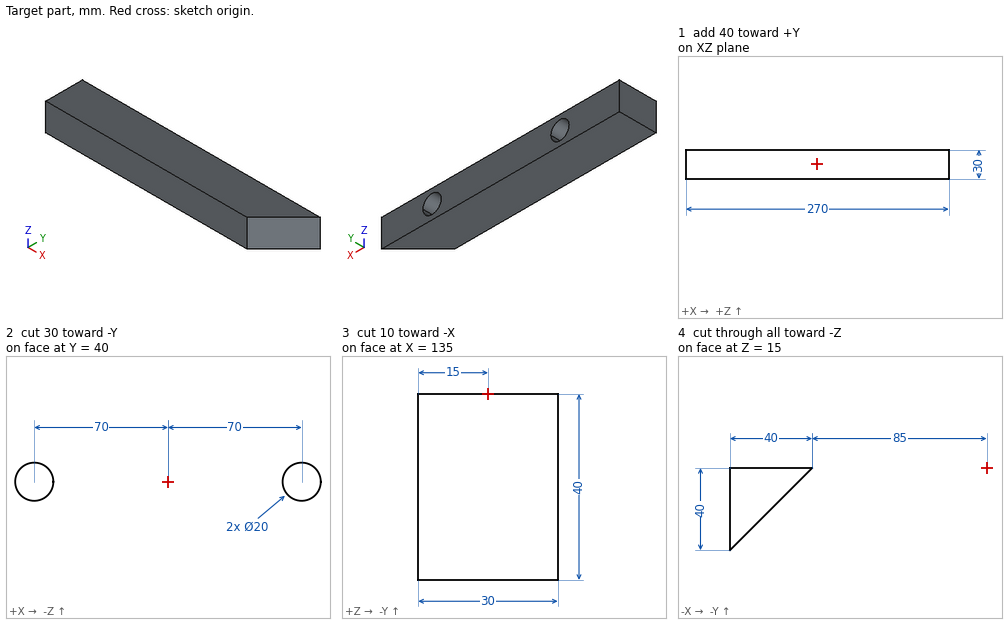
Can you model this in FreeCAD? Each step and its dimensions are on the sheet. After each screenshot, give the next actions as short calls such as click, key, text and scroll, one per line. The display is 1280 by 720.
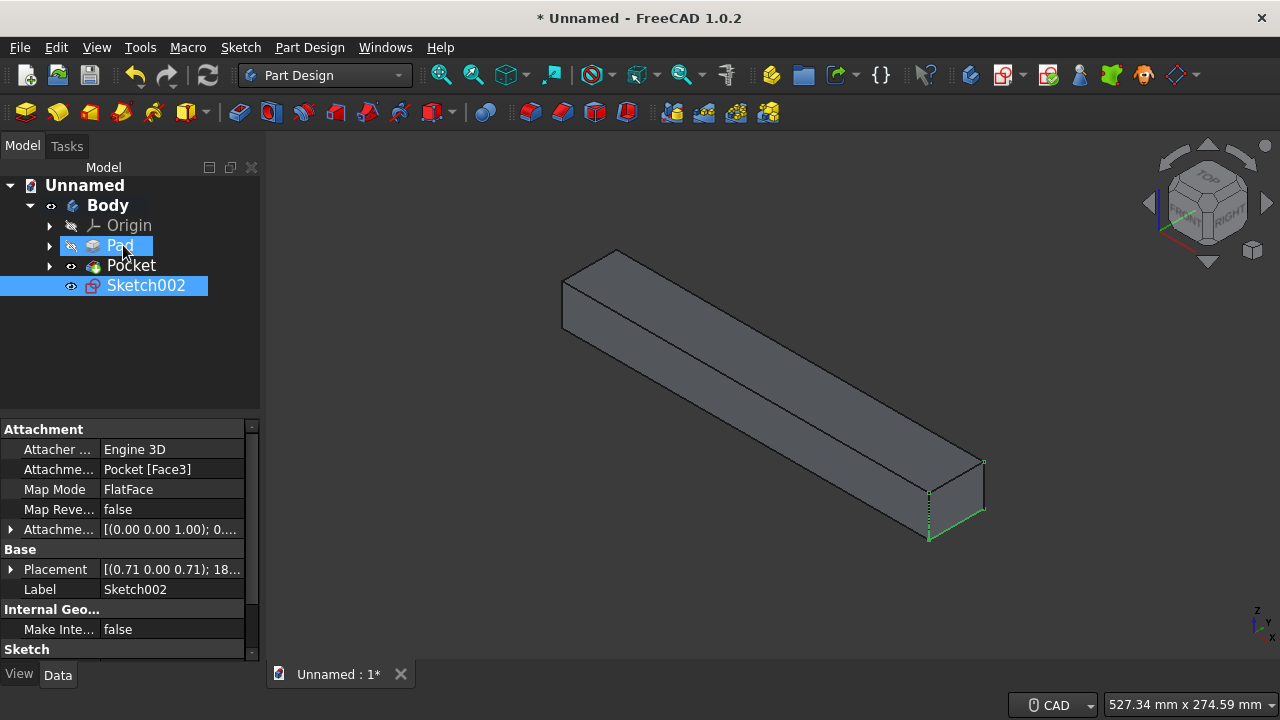
click(240, 112)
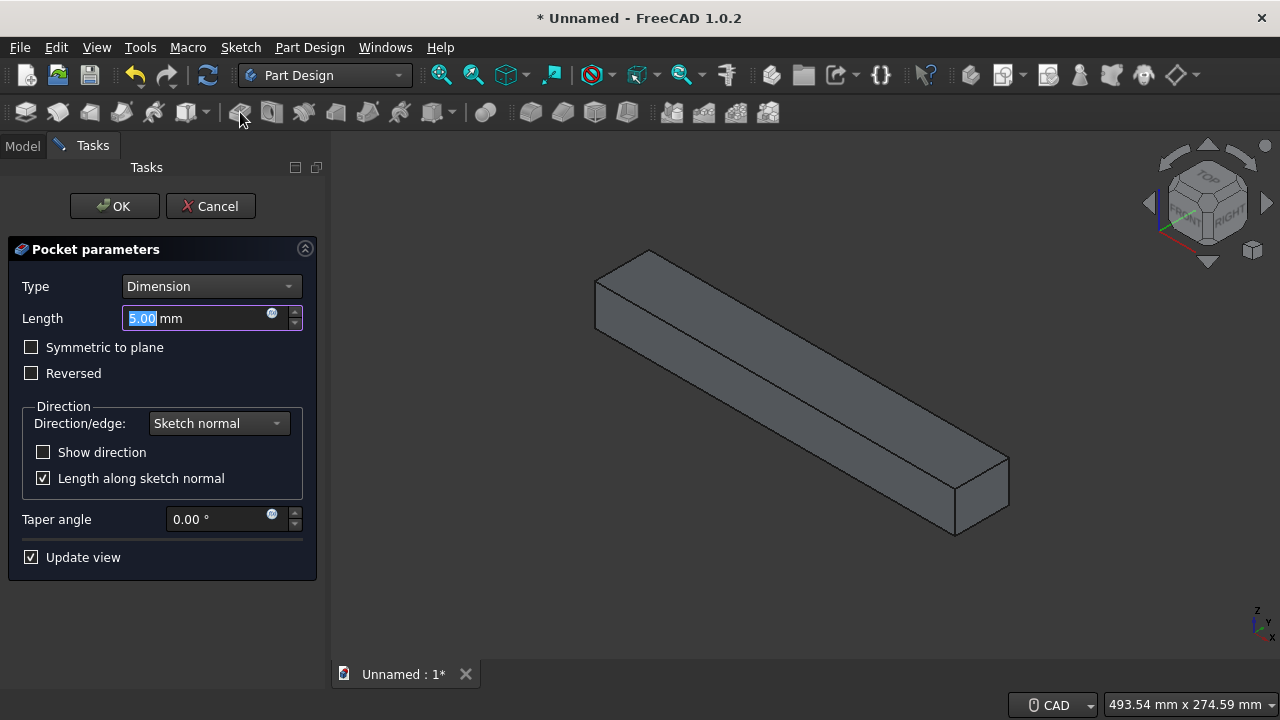
text(10)
key(Tab)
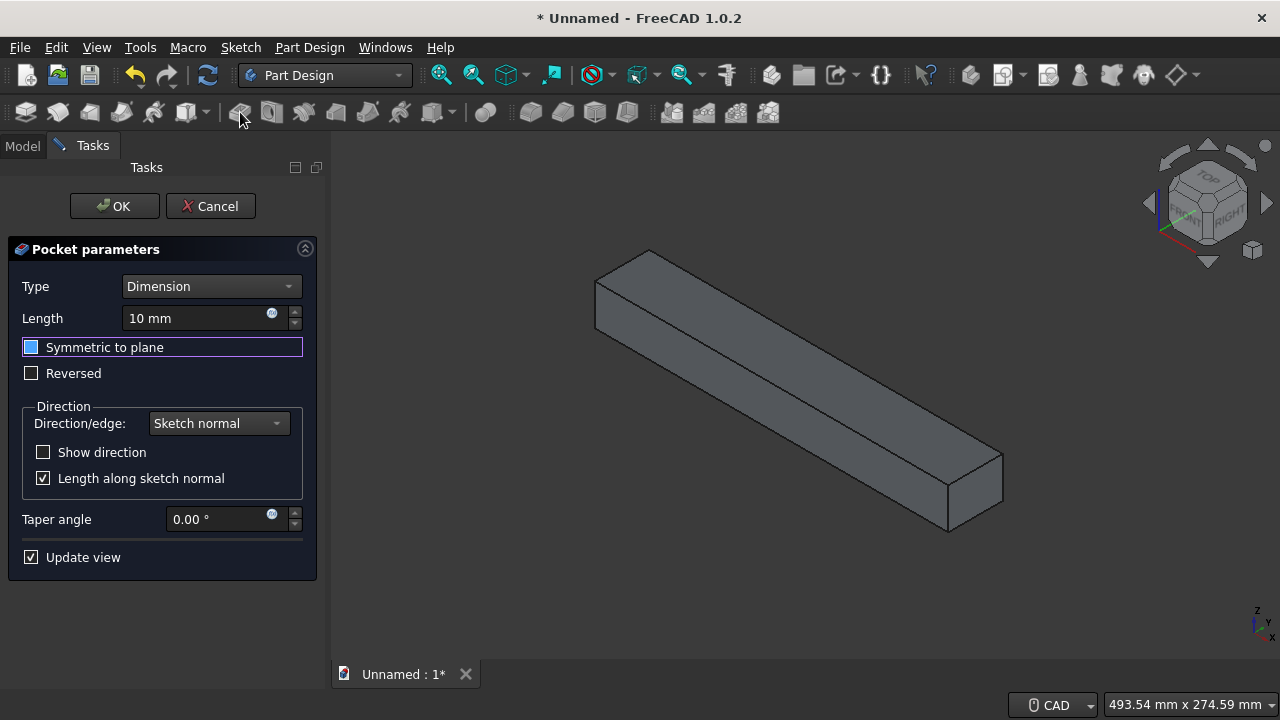
click(115, 206)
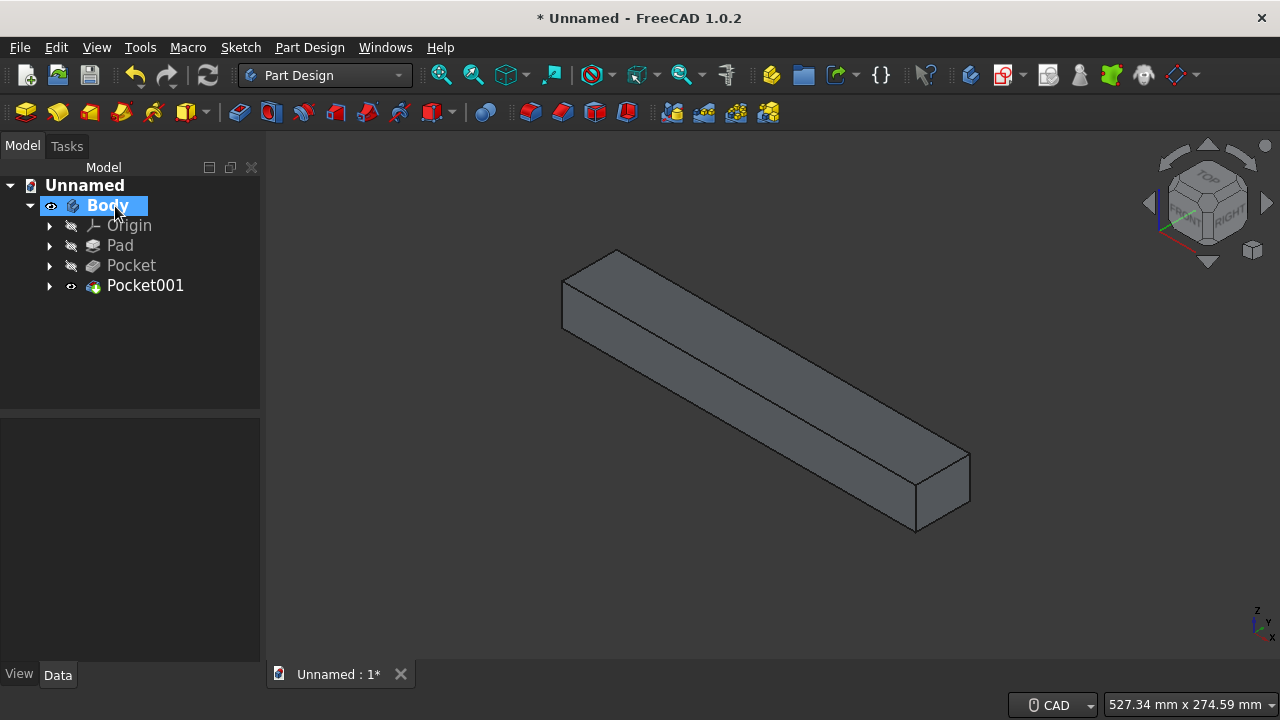
click(867, 425)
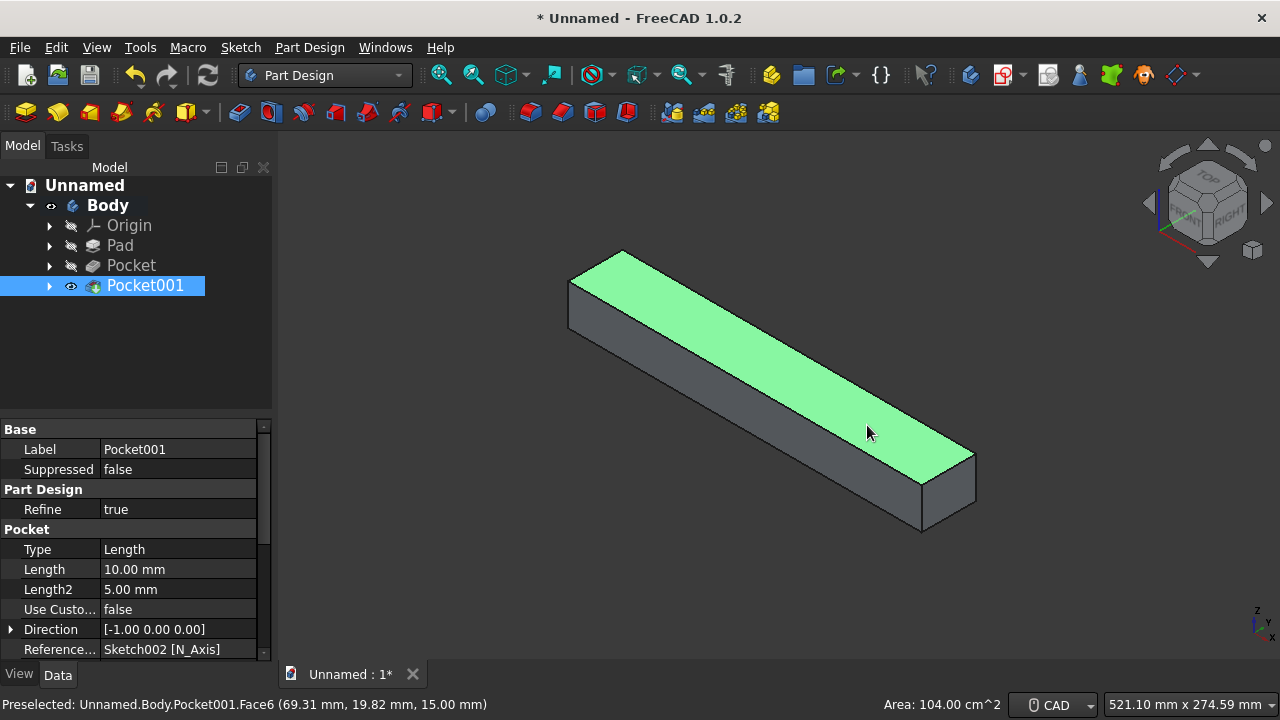
click(1004, 76)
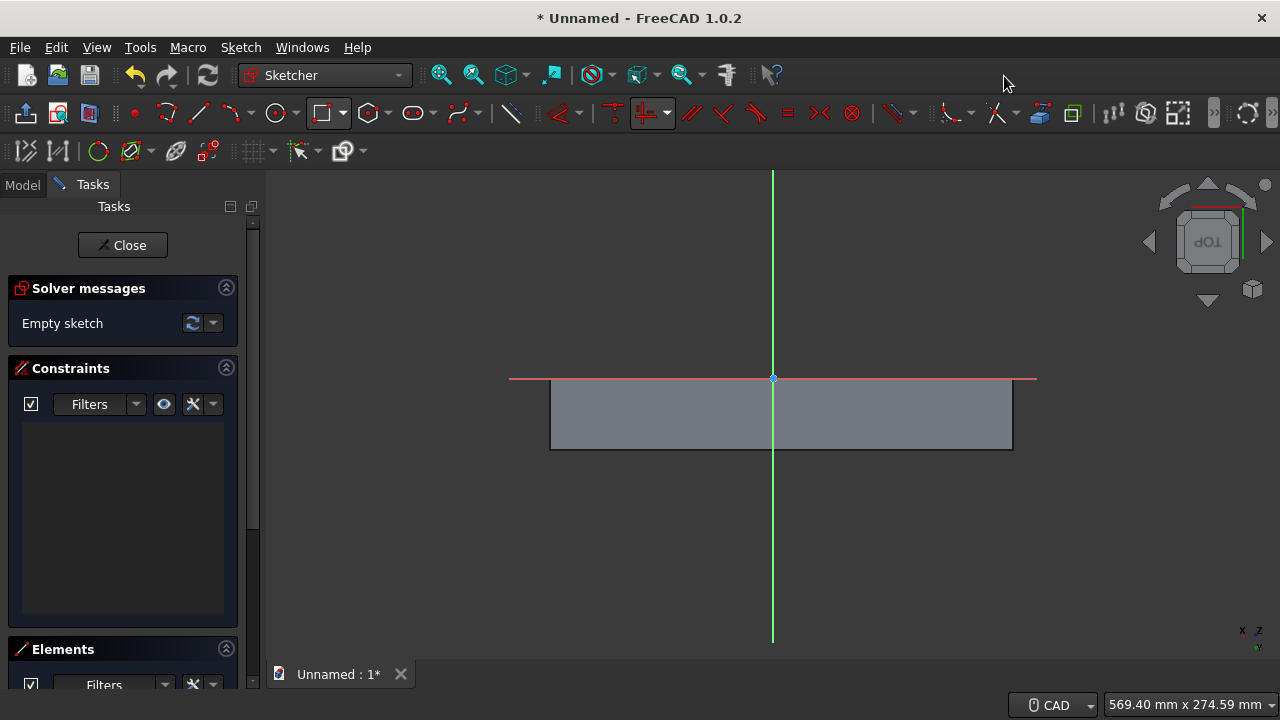
scroll(547, 415, up, 7)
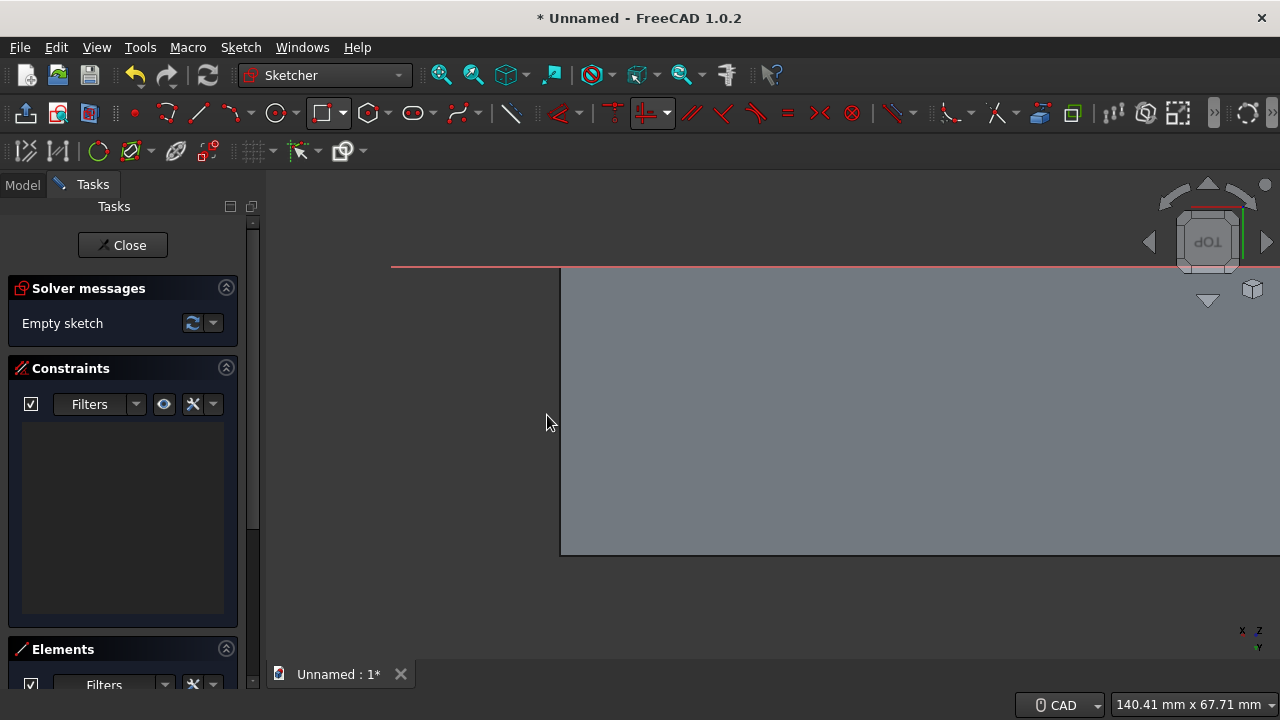
click(168, 114)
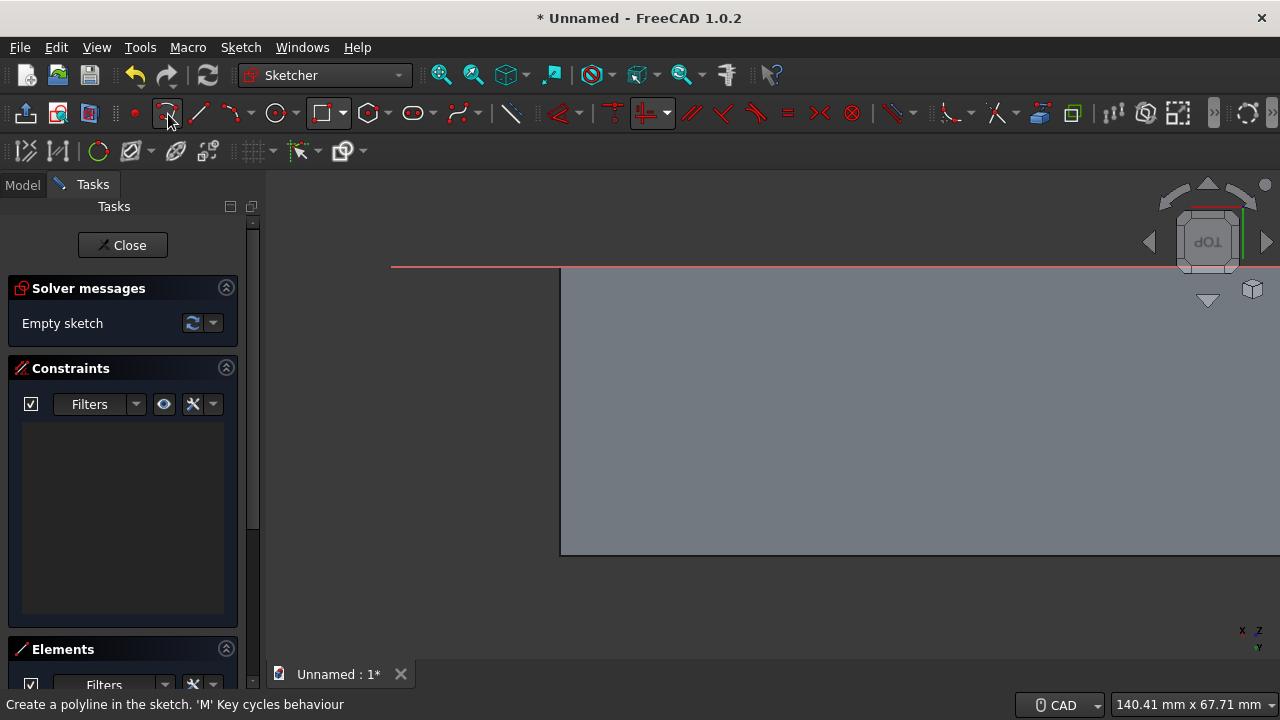
click(849, 267)
click(560, 276)
click(560, 556)
click(849, 267)
key(Escape)
key(Escape)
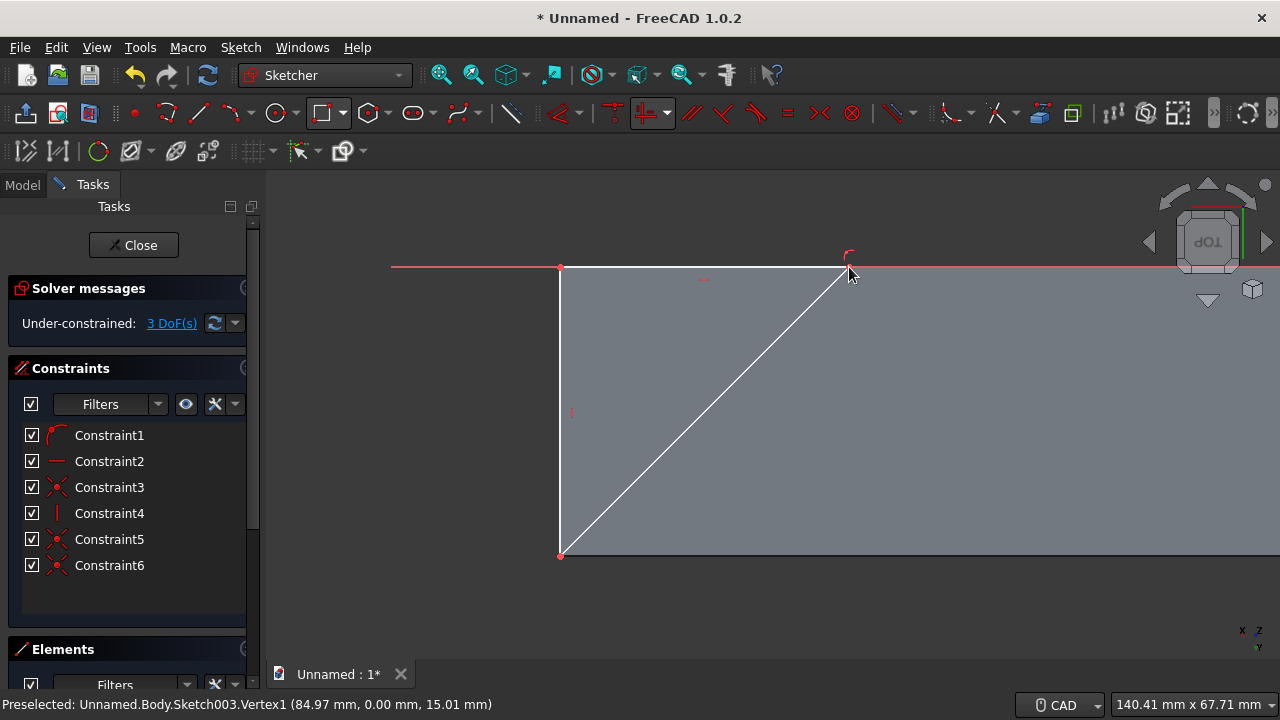
click(558, 114)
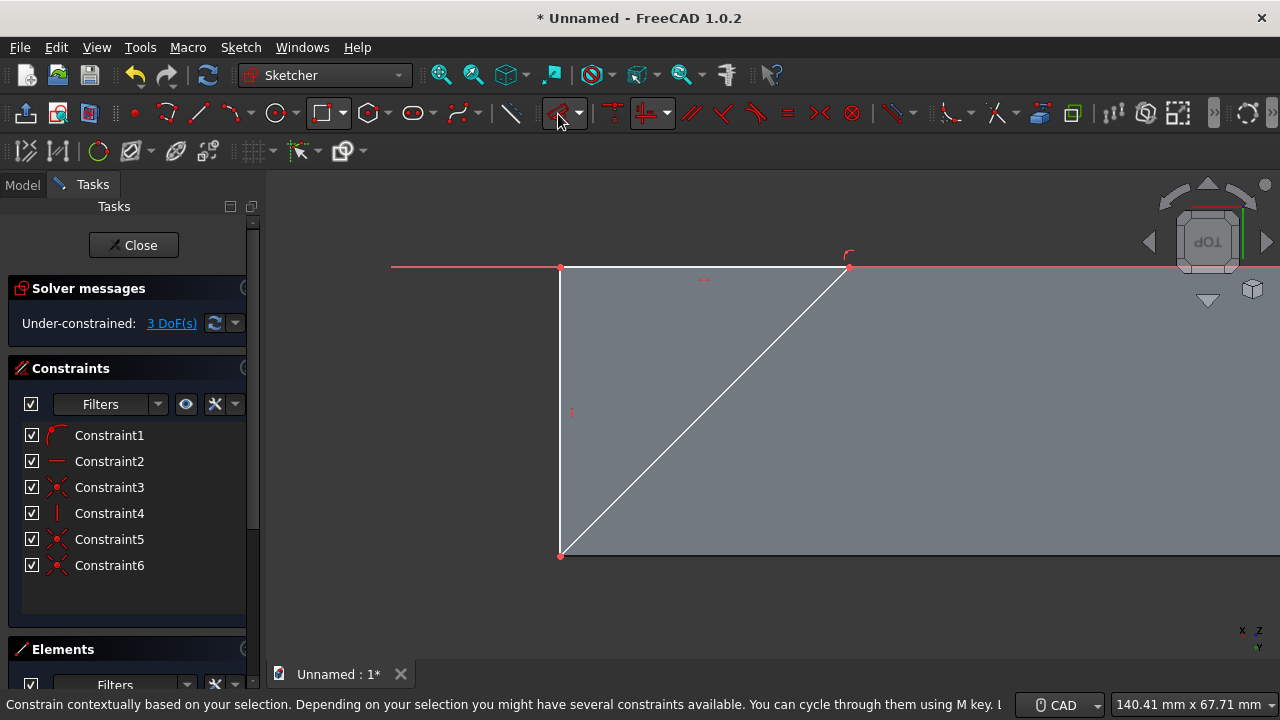
click(762, 267)
click(705, 233)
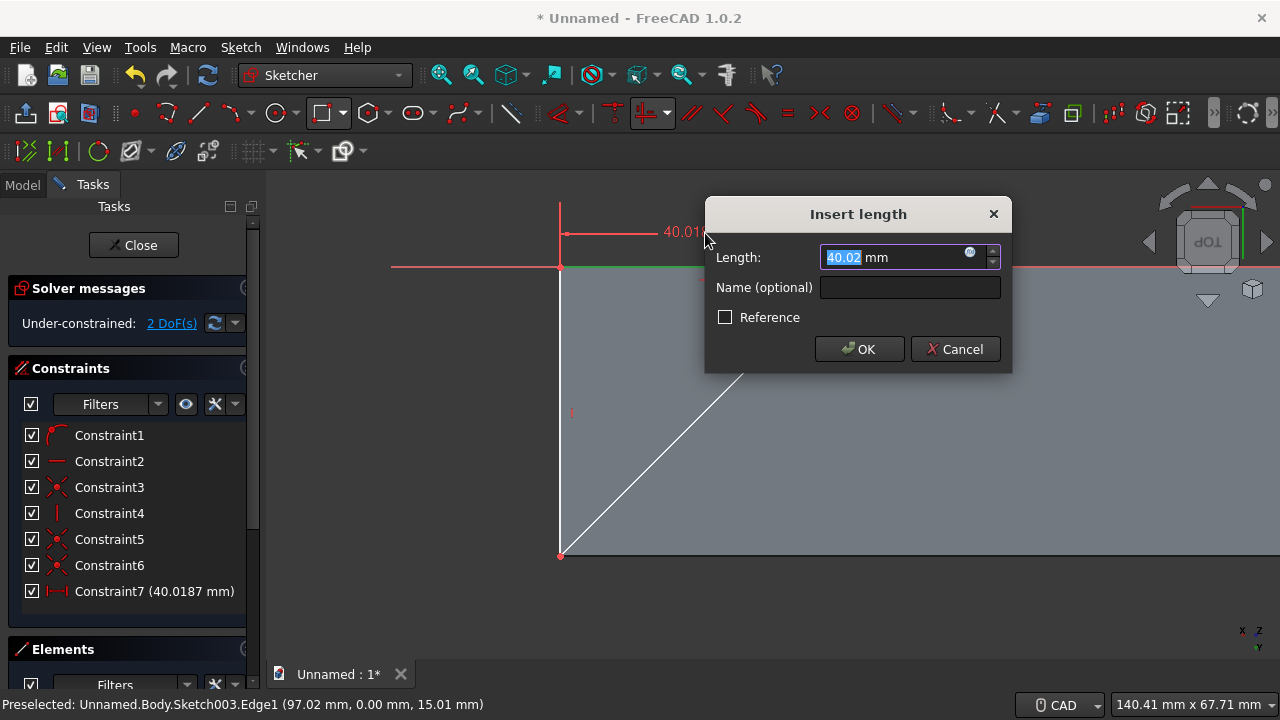
text(40)
key(Return)